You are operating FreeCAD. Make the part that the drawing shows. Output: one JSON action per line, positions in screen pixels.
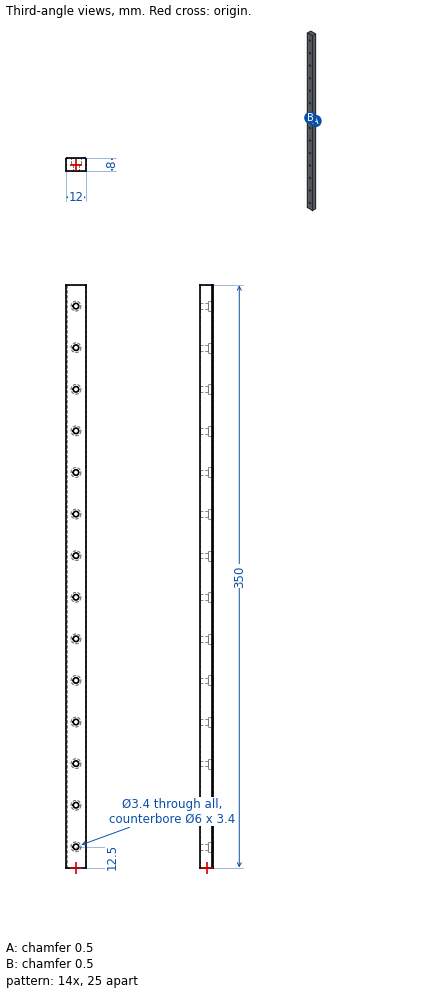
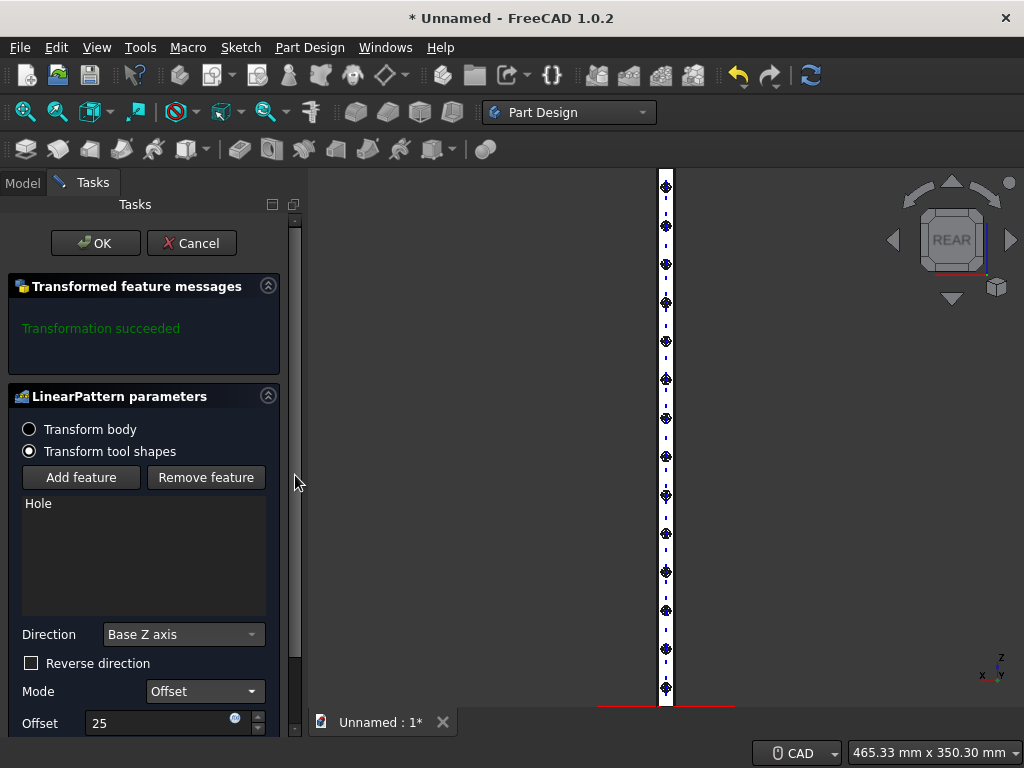
{"action": "left_click", "coordinate": [96, 243]}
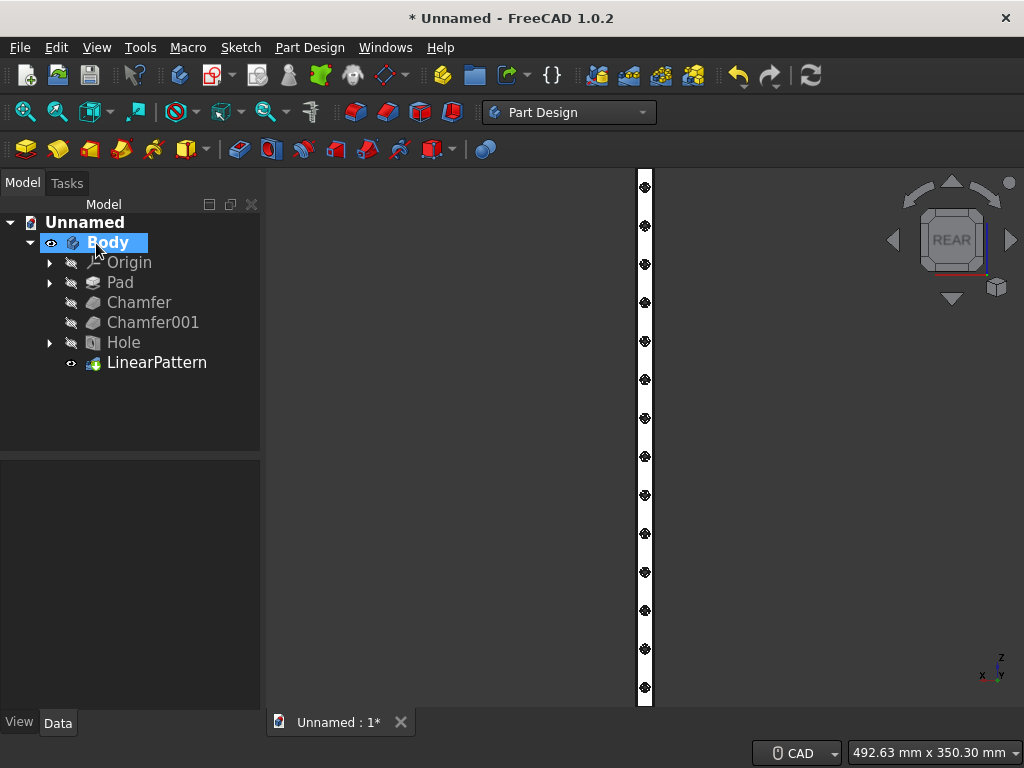
{"action": "key", "text": "0"}